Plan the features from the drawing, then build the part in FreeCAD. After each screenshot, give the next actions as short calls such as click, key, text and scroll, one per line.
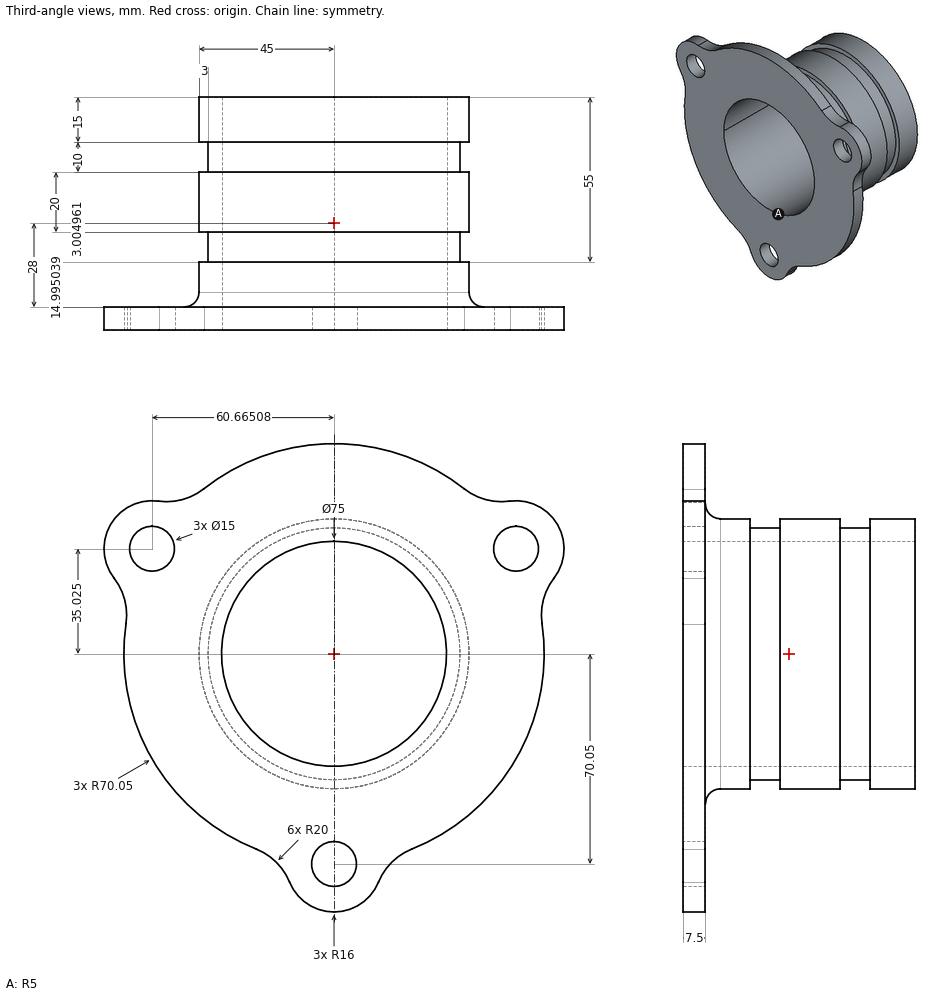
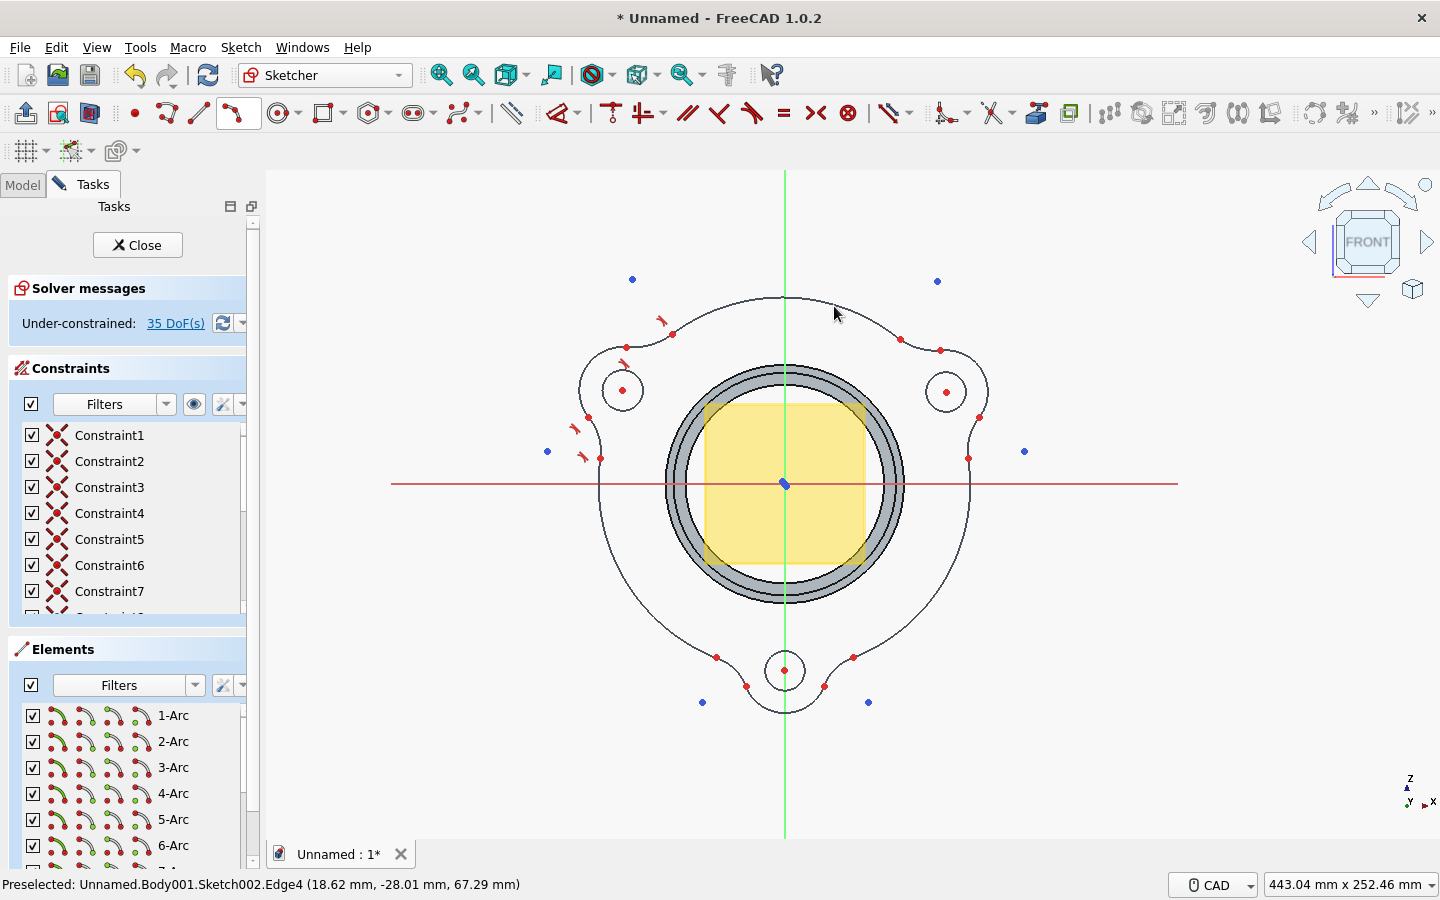
click(836, 305)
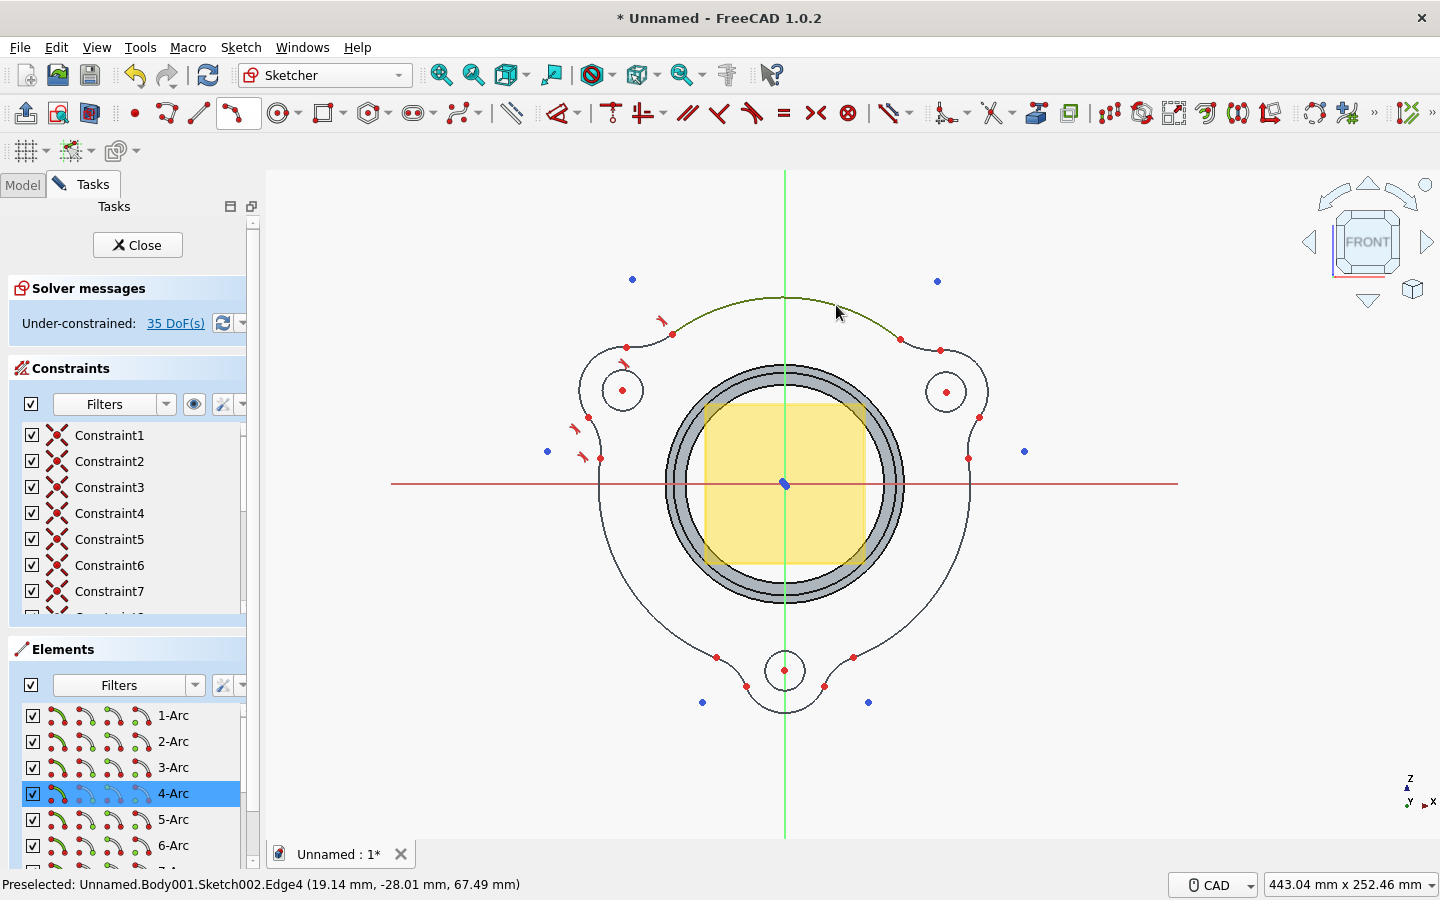
click(911, 346)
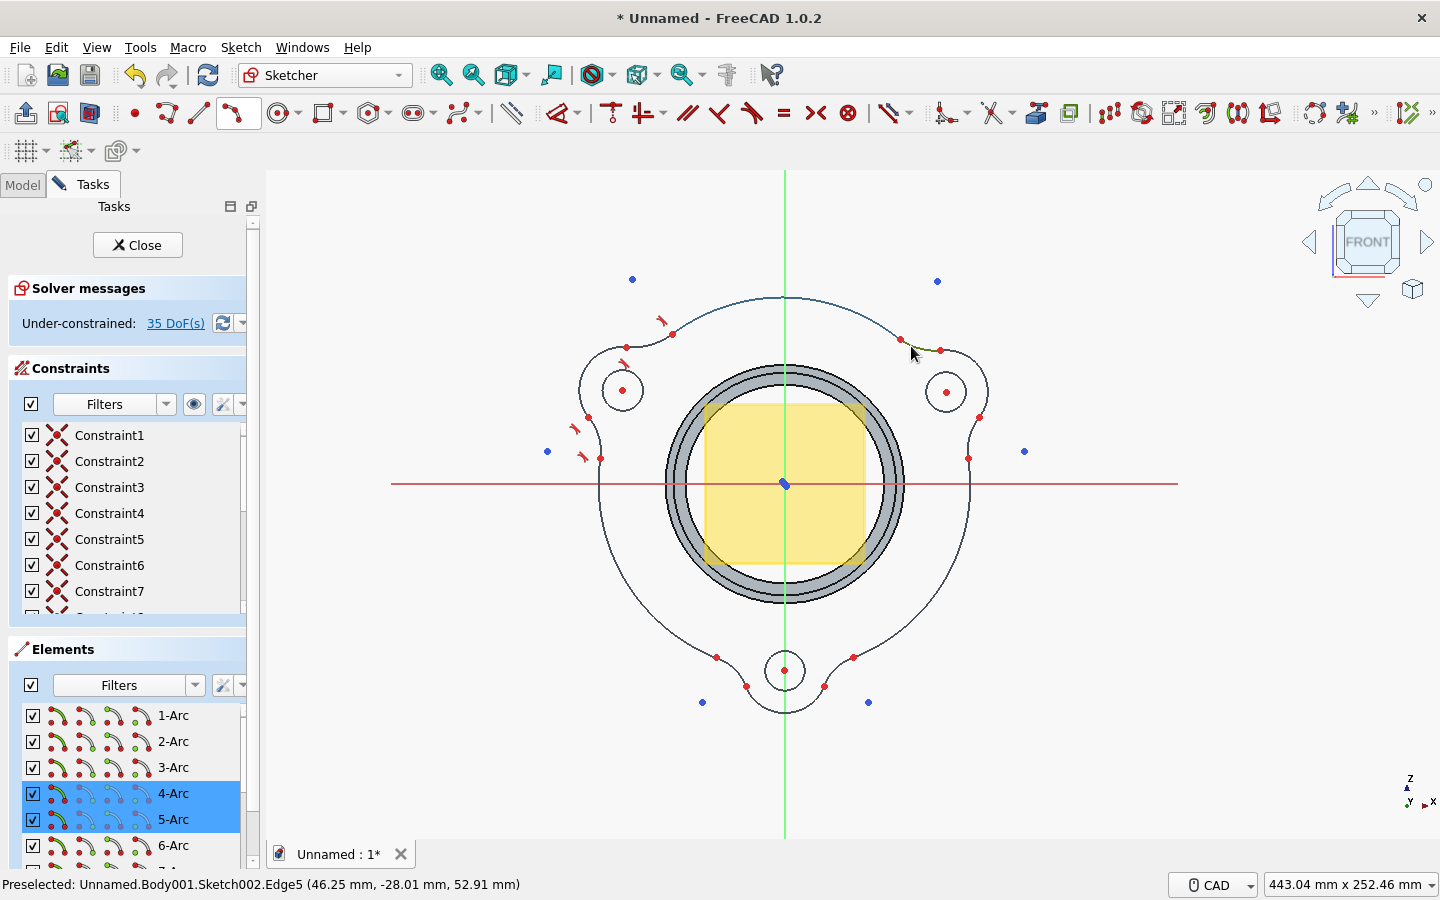
click(752, 114)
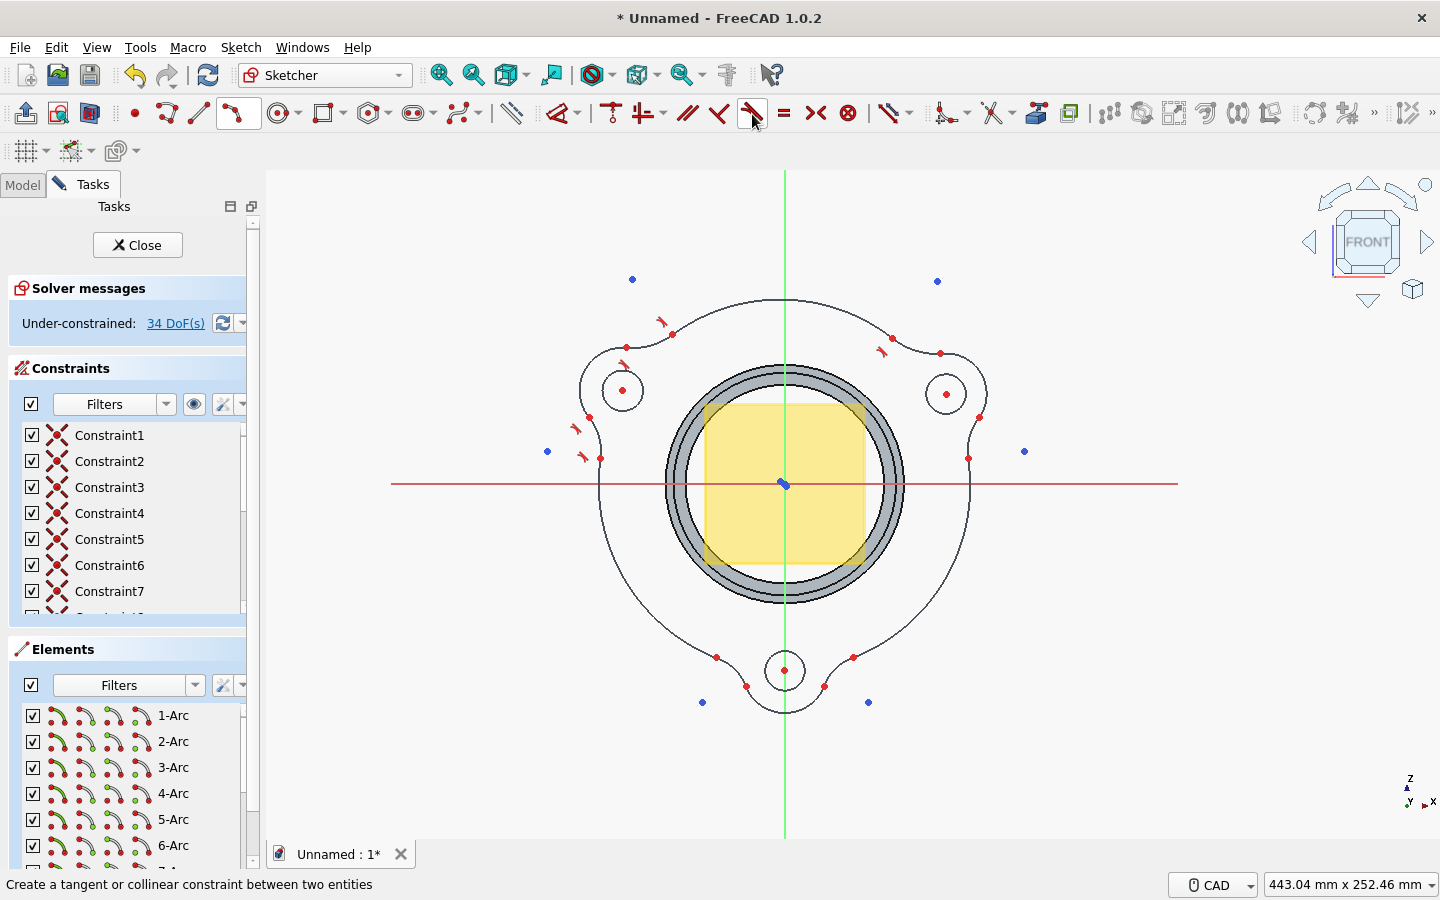
click(906, 347)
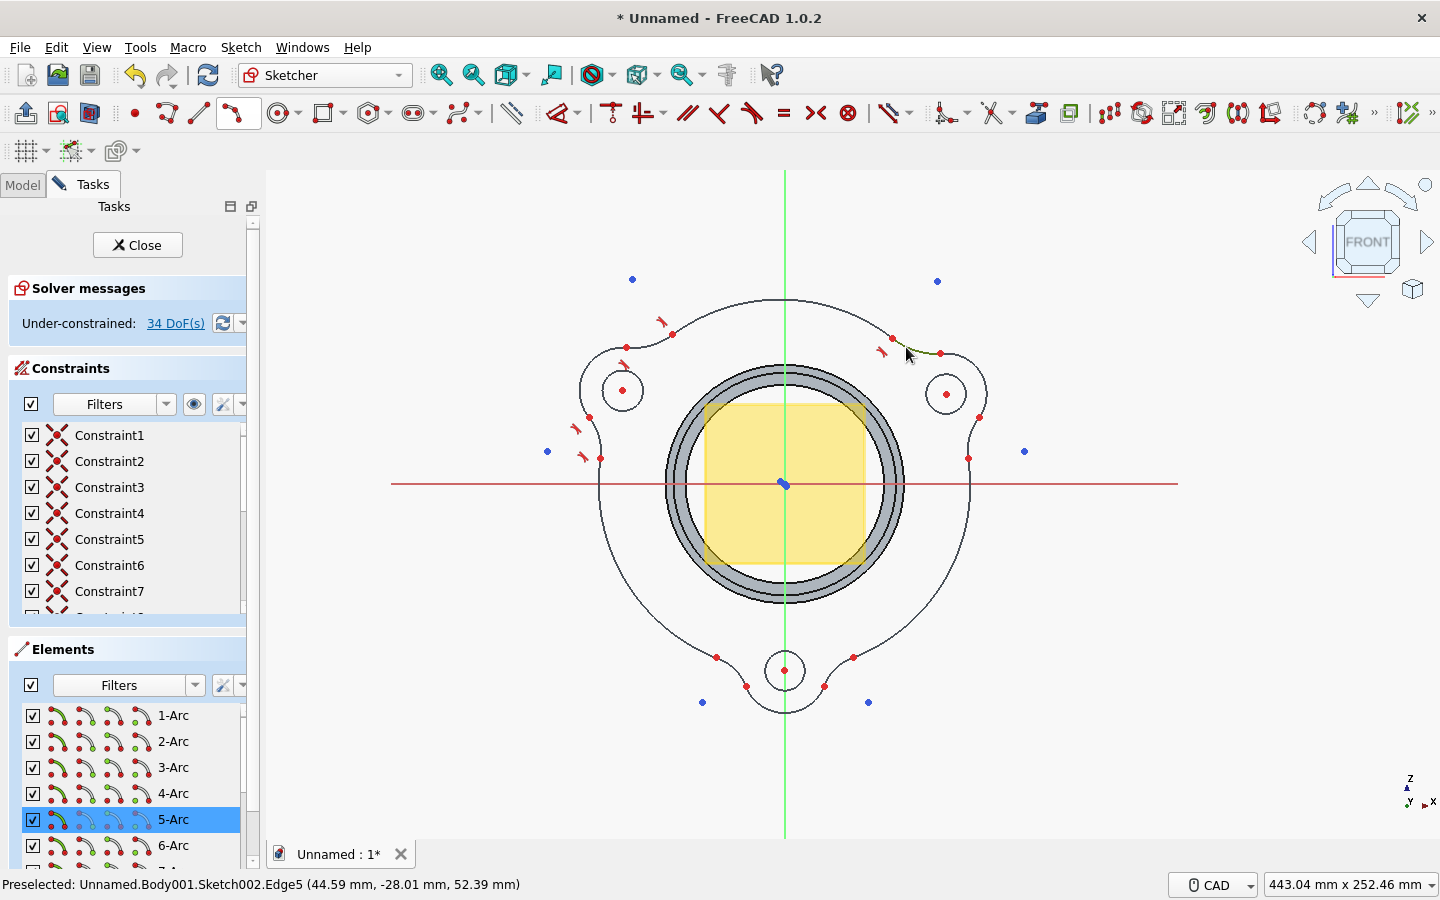
click(987, 391)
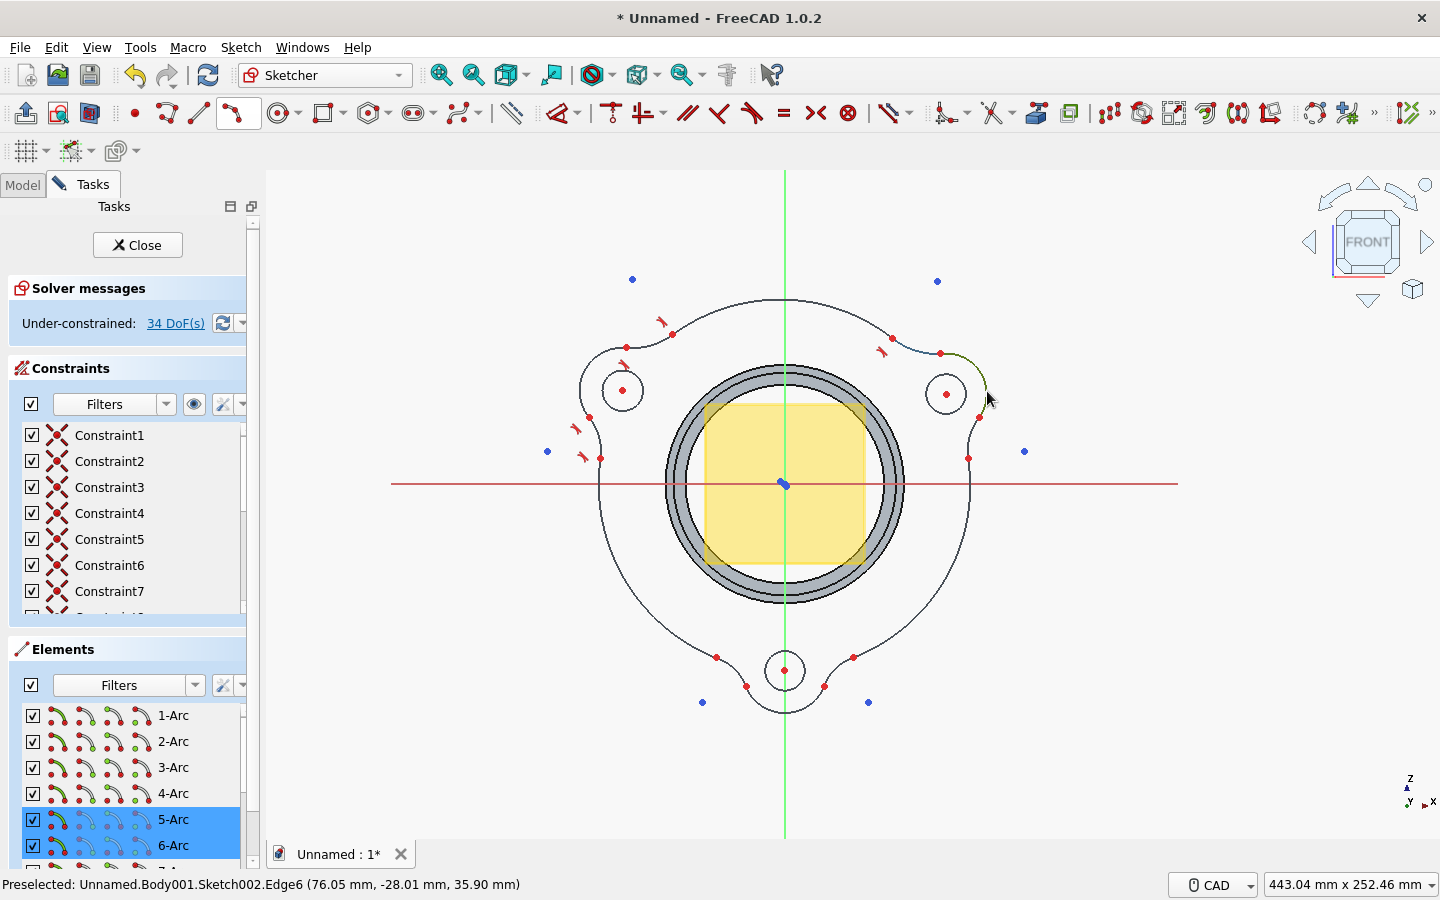
key(t)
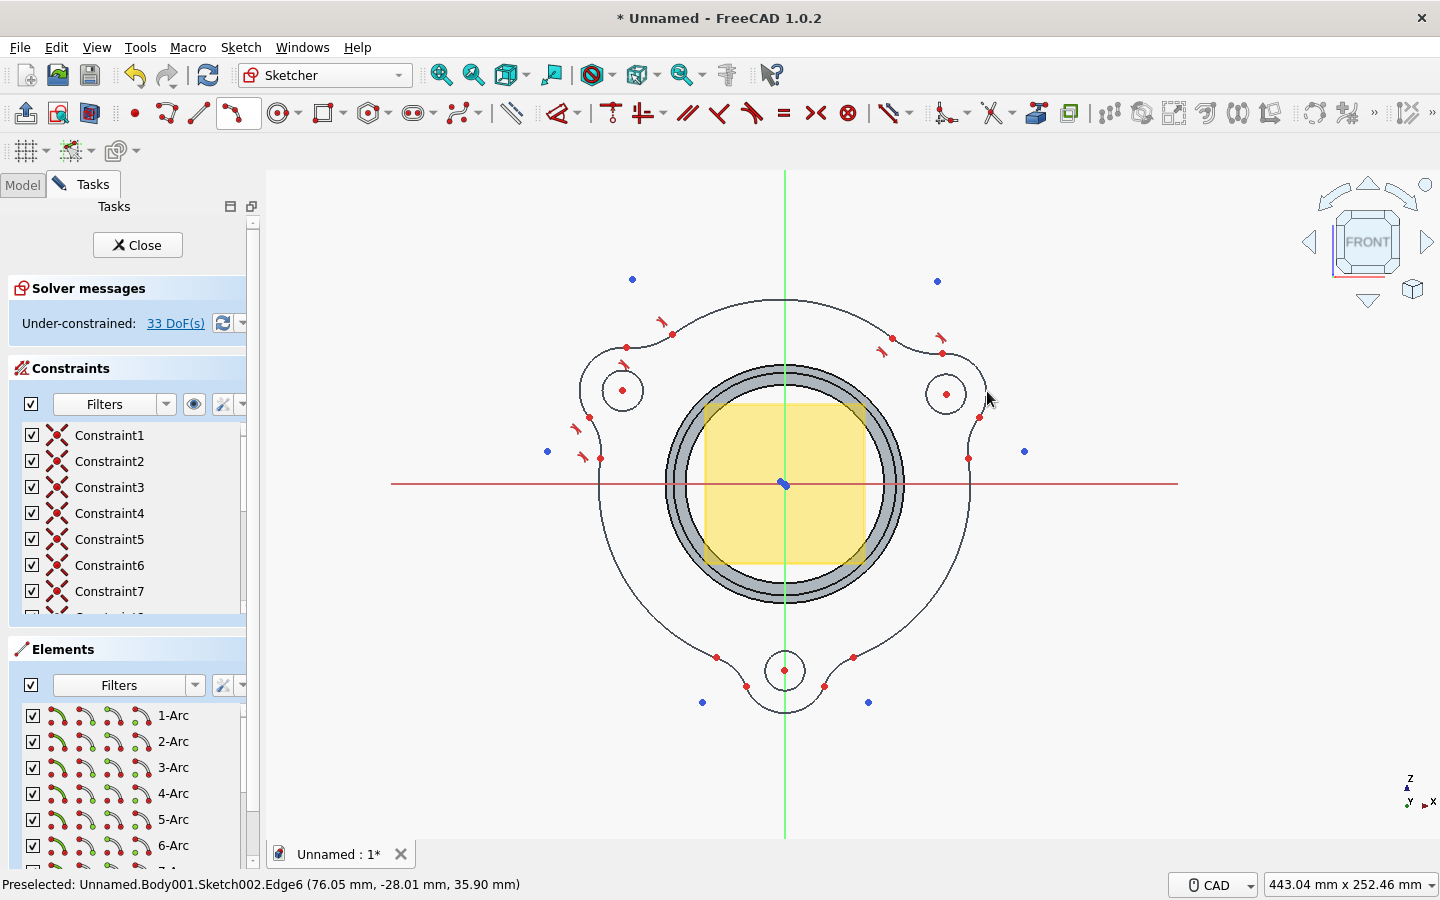
click(987, 392)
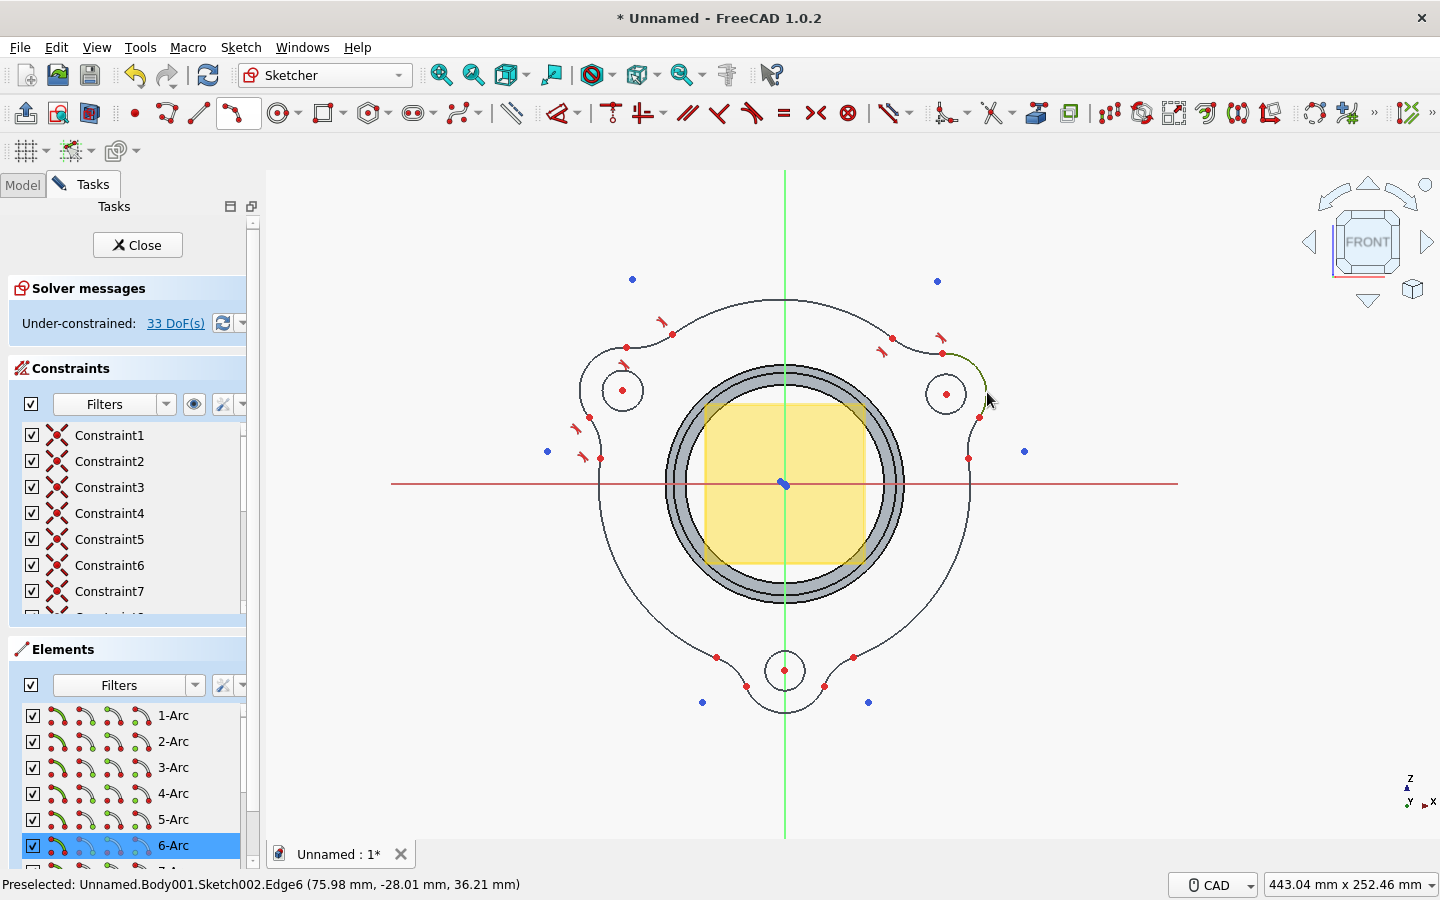
click(972, 429)